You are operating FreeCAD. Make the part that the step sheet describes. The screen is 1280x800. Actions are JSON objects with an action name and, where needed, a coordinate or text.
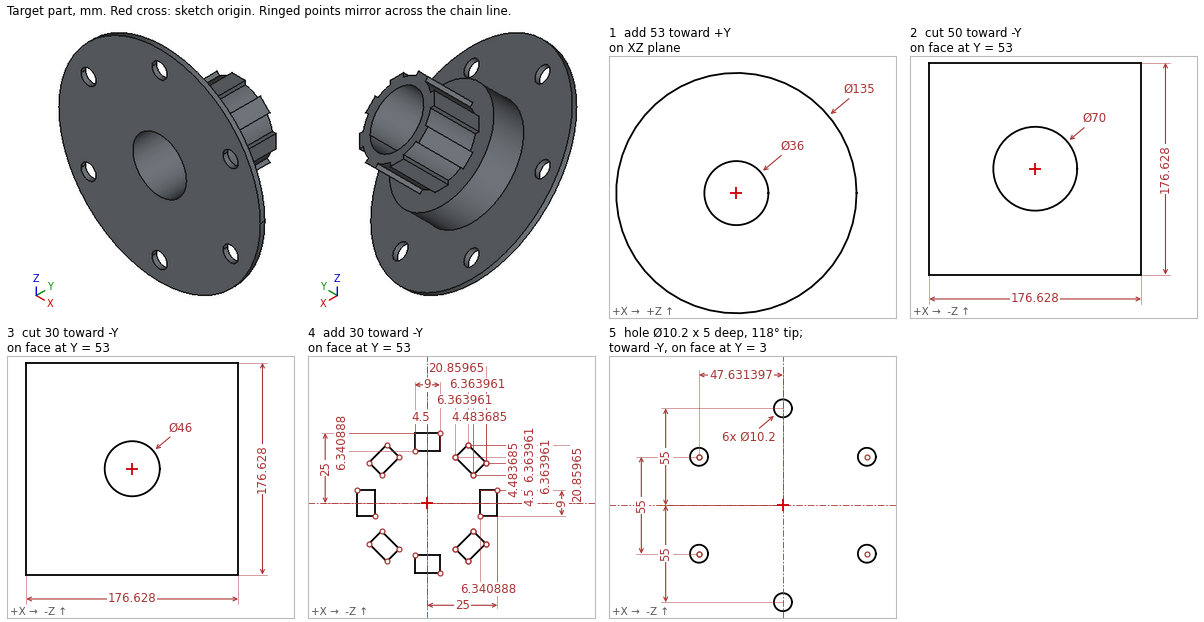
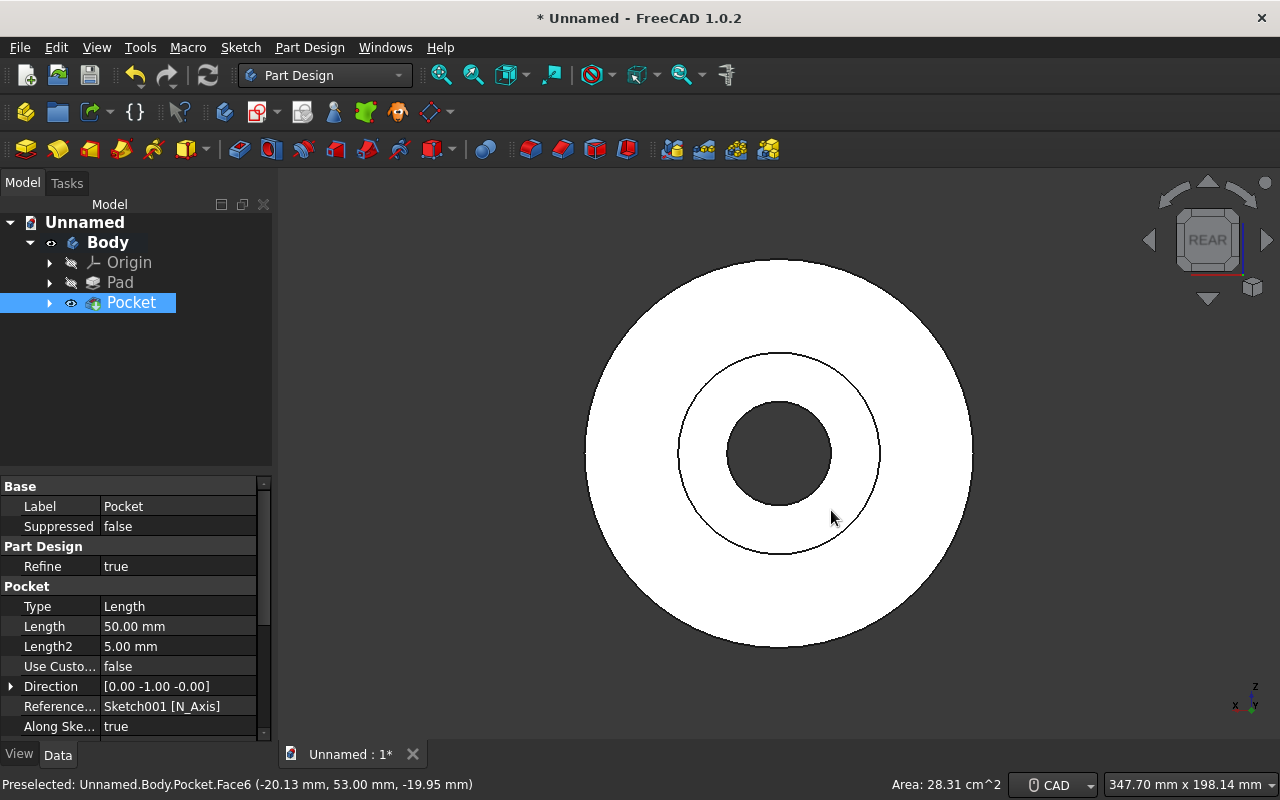
{"action": "left_click", "coordinate": [258, 112]}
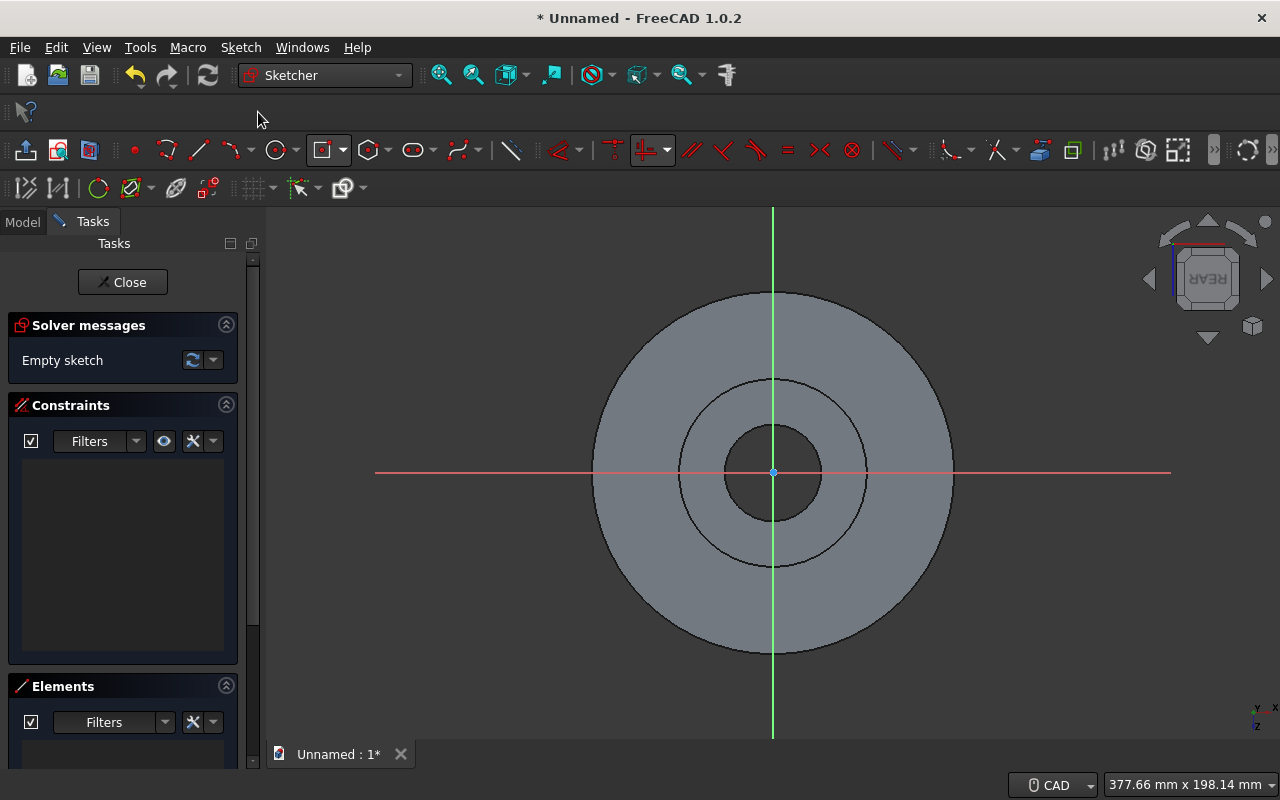
{"action": "scroll", "coordinate": [565, 473], "scroll_direction": "down", "scroll_amount": 2}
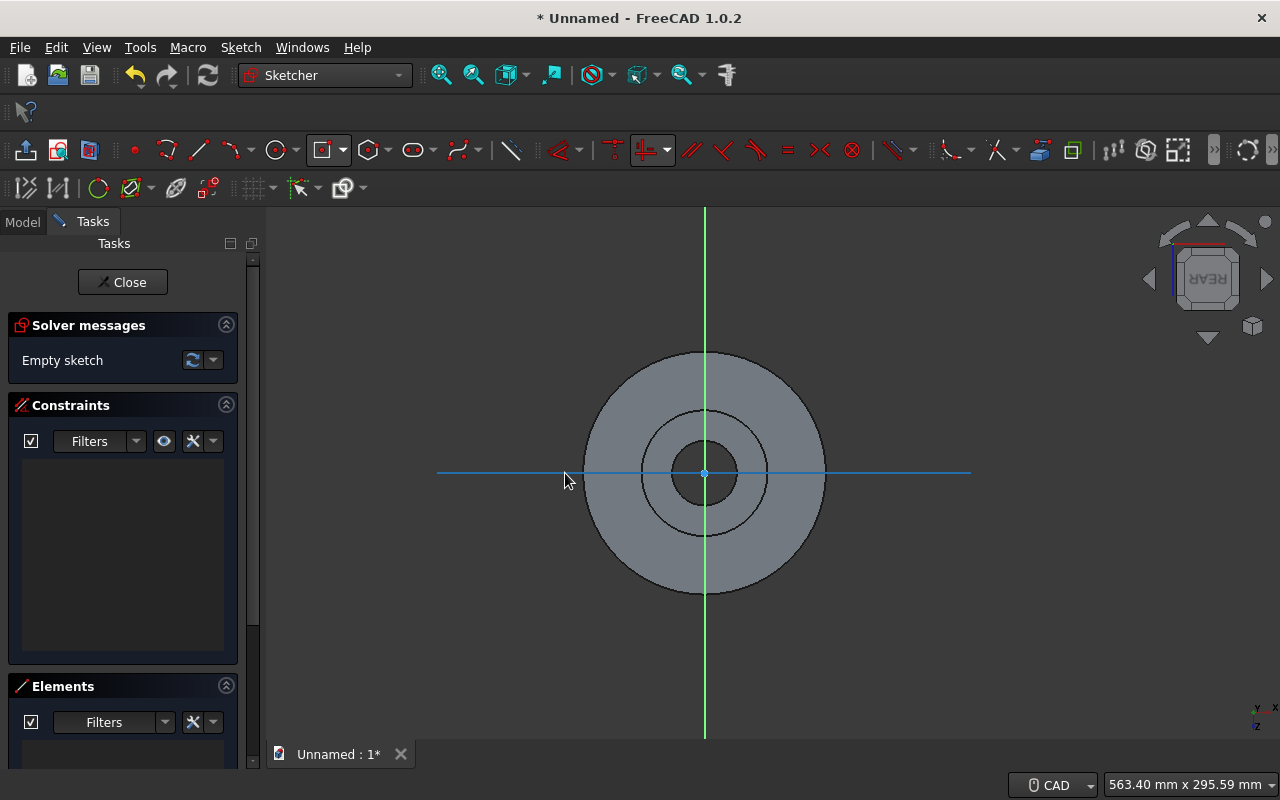
{"action": "left_click", "coordinate": [322, 150]}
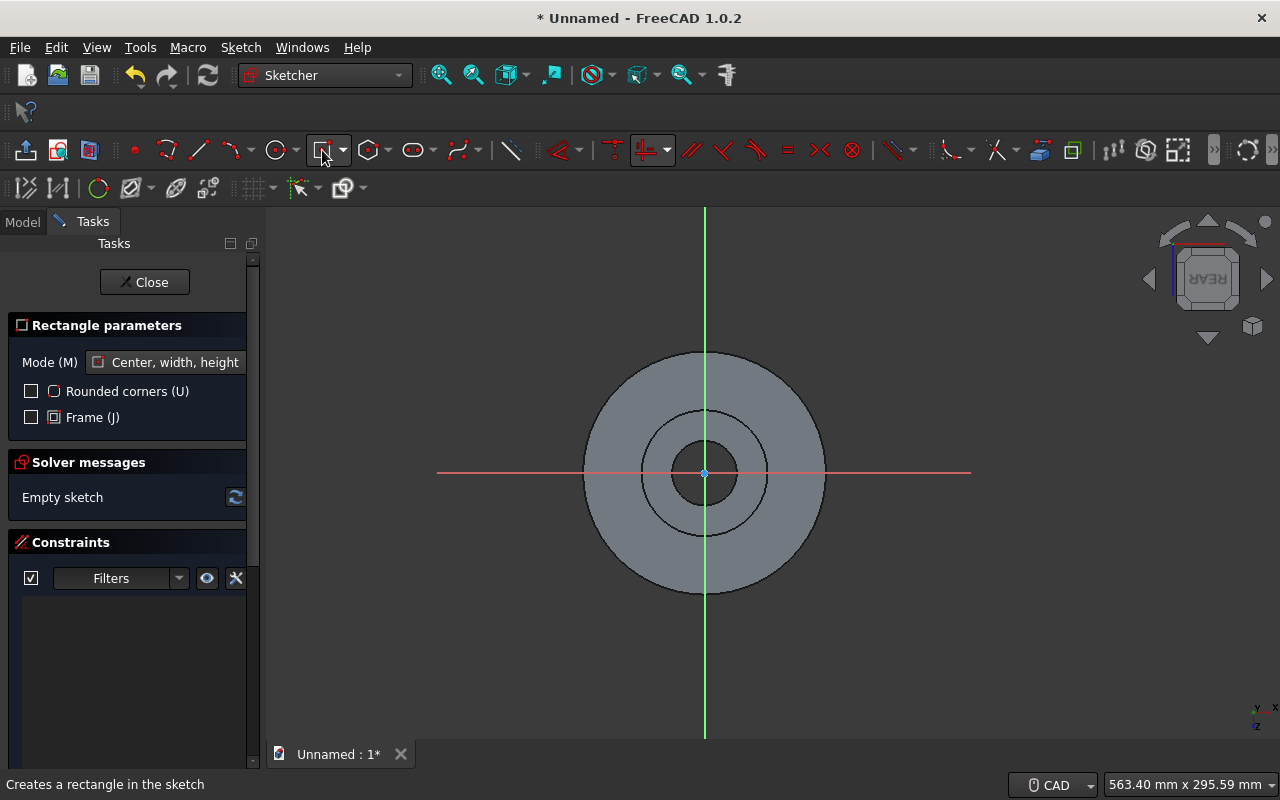
{"action": "left_click", "coordinate": [705, 473]}
{"action": "left_click", "coordinate": [863, 314]}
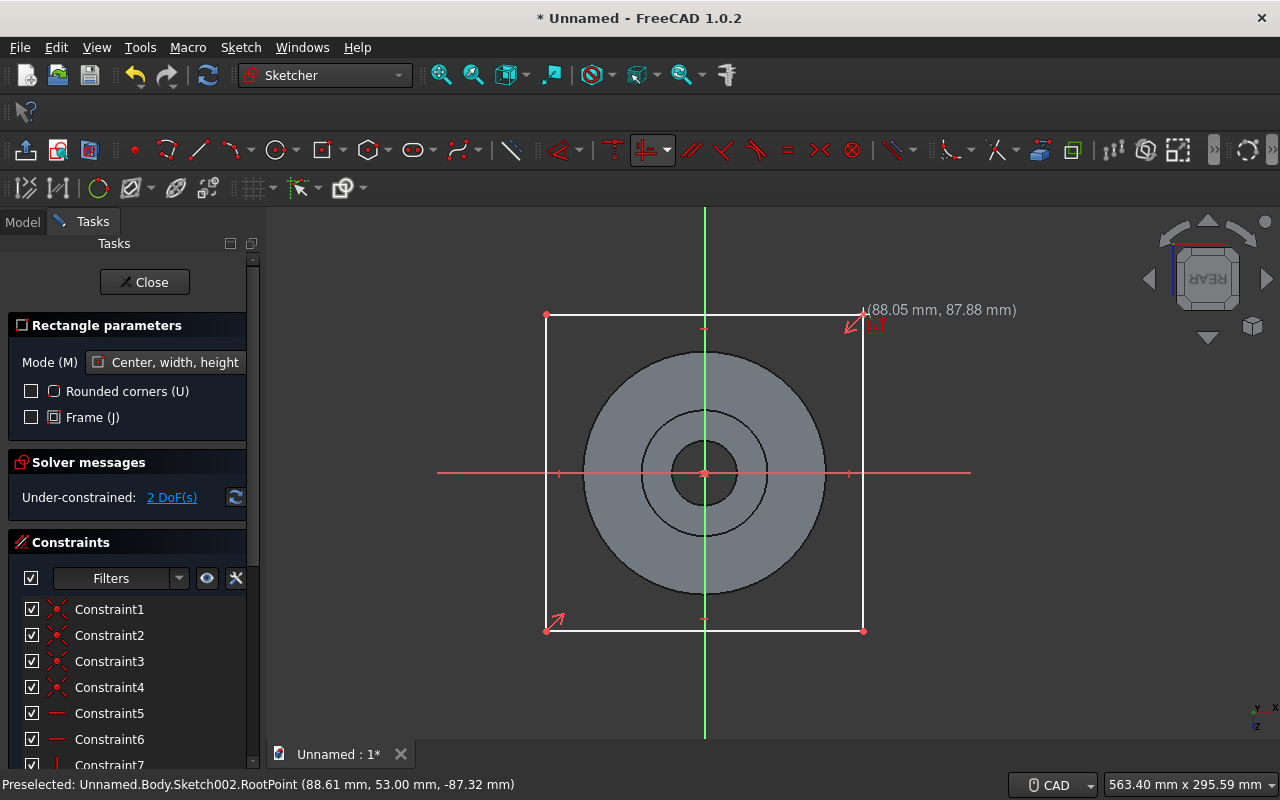
{"action": "left_click", "coordinate": [276, 150]}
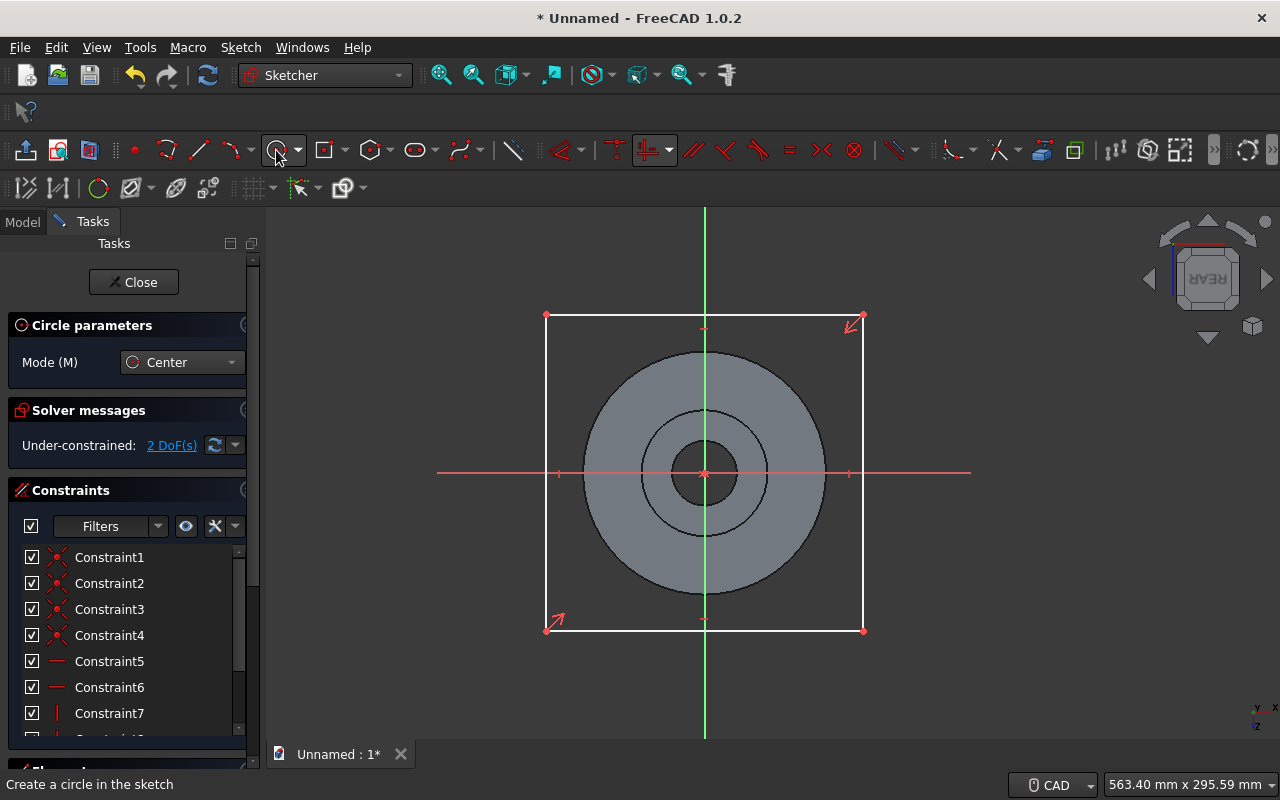
{"action": "left_click", "coordinate": [705, 473]}
{"action": "left_click", "coordinate": [734, 444]}
{"action": "key", "text": "Escape"}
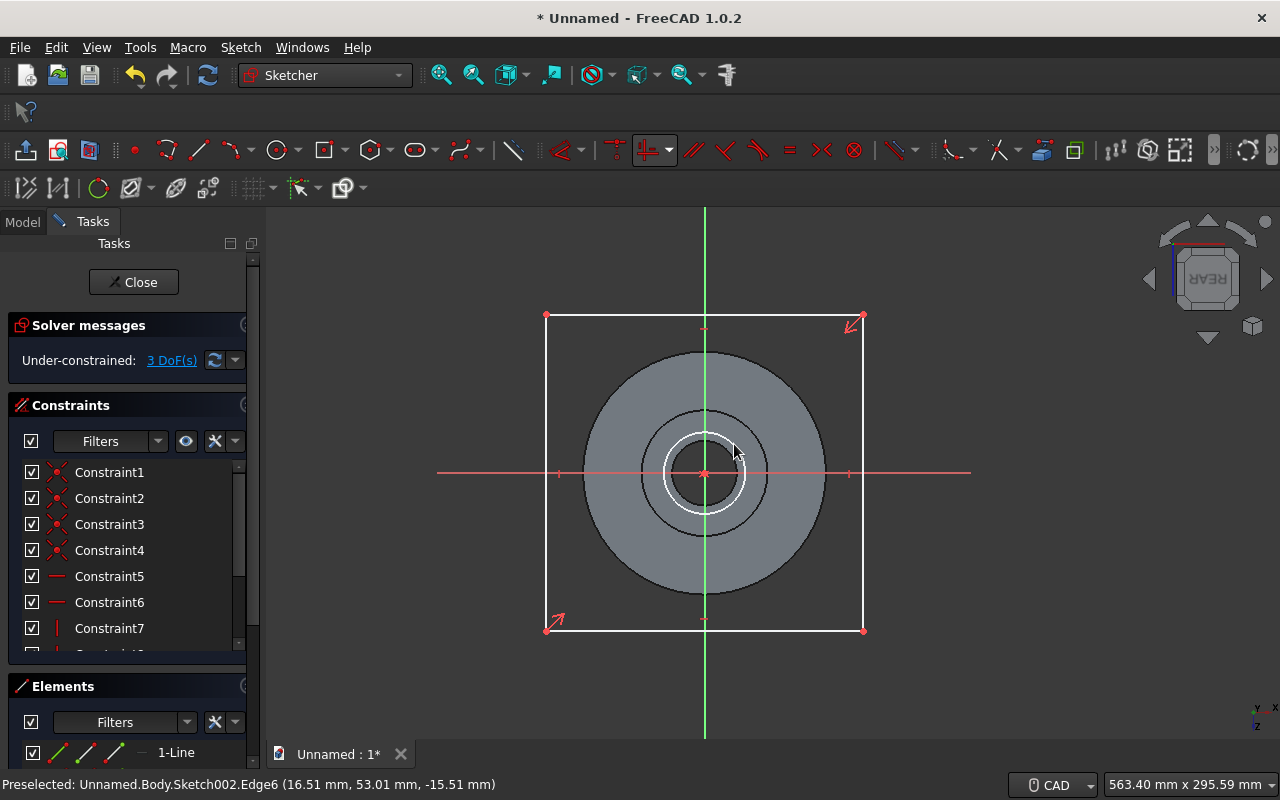
{"action": "left_click", "coordinate": [560, 150]}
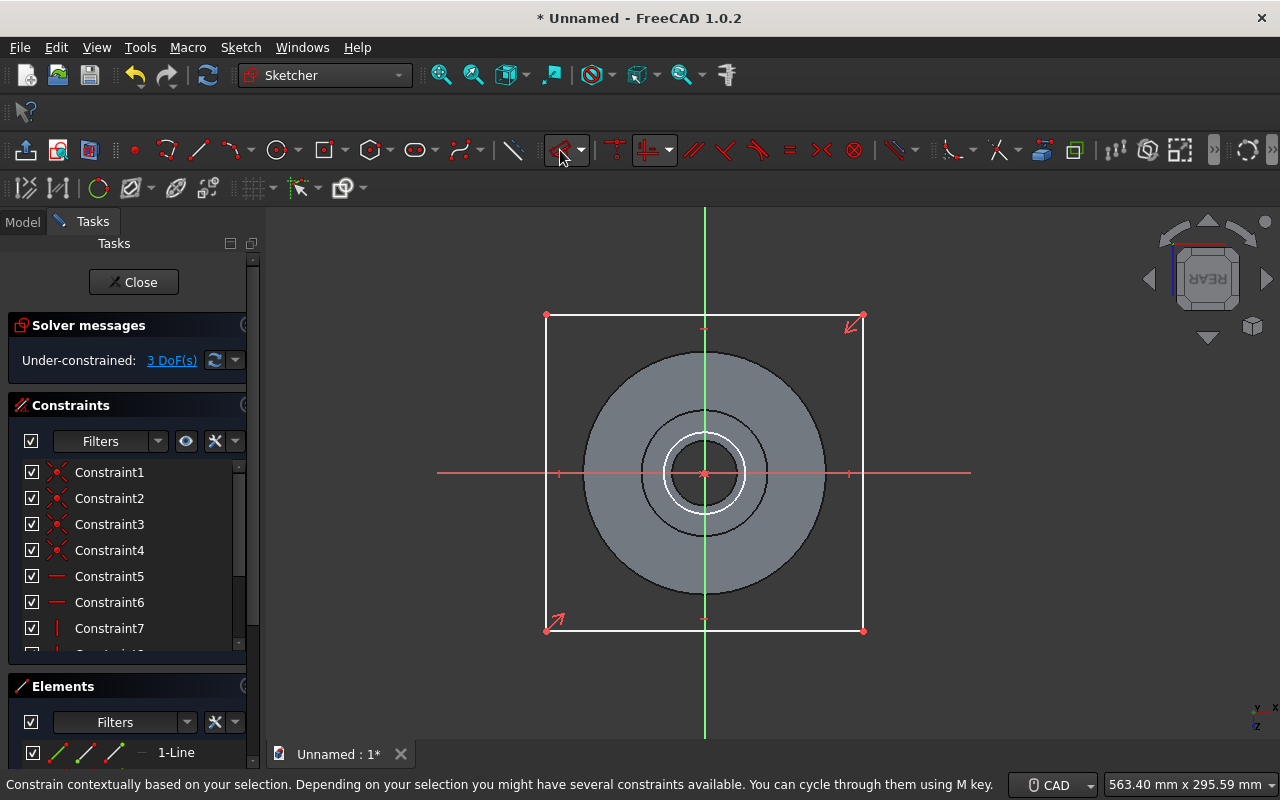
{"action": "left_click", "coordinate": [733, 444]}
{"action": "left_click", "coordinate": [755, 421]}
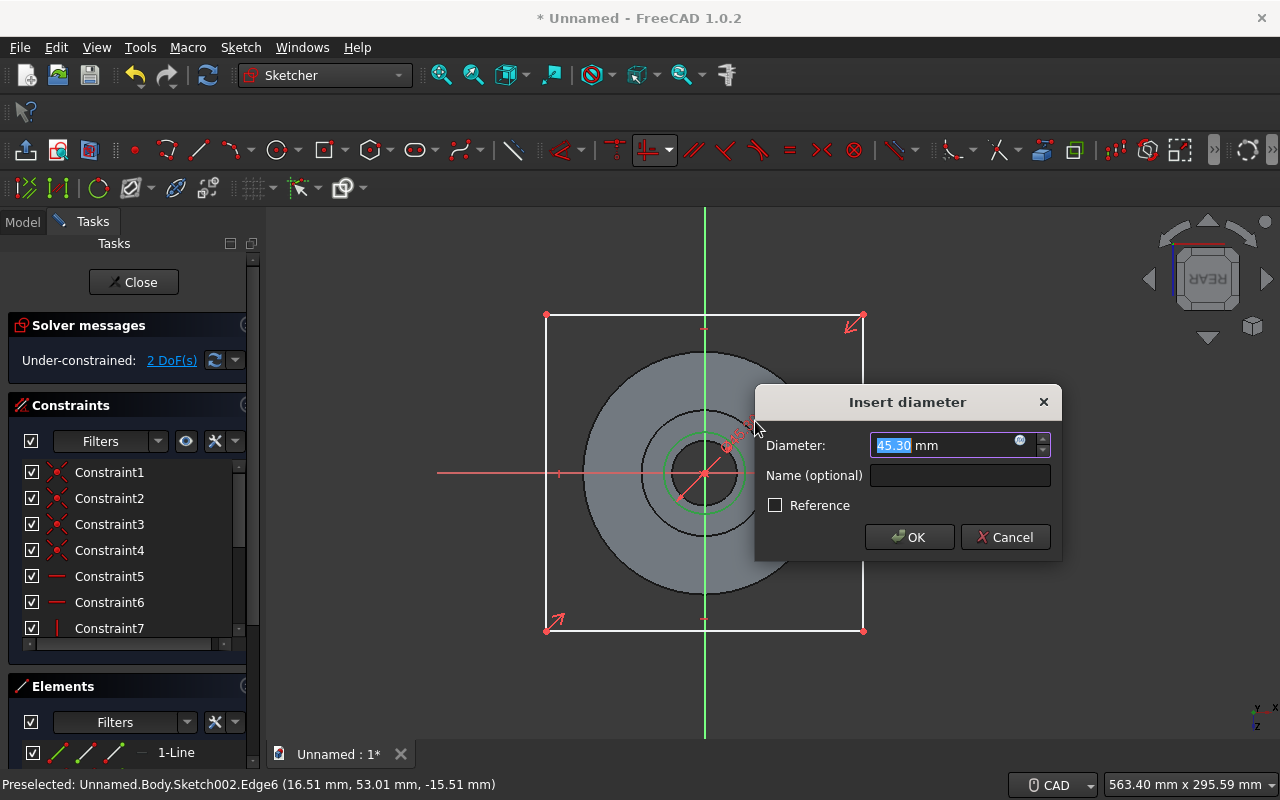
{"action": "type", "text": "46"}
{"action": "key", "text": "Return"}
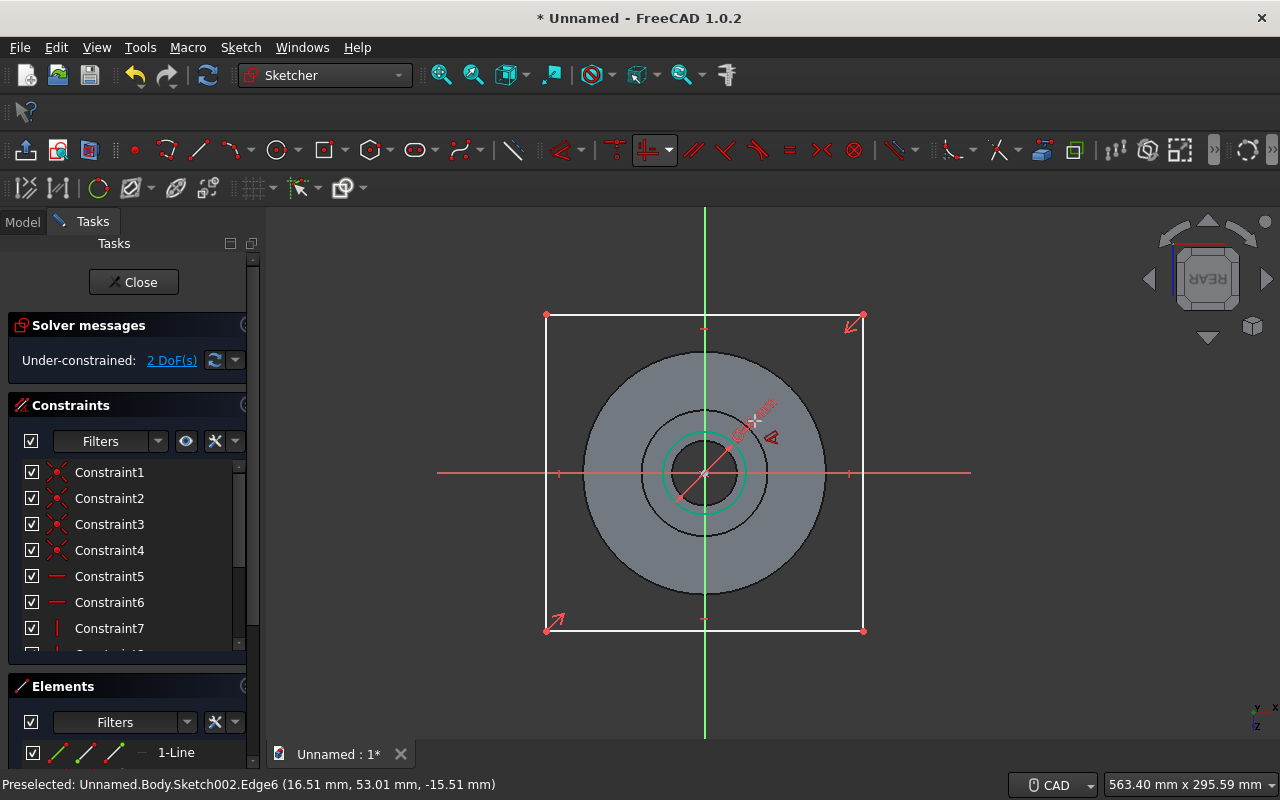
{"action": "left_click", "coordinate": [641, 631]}
{"action": "left_click", "coordinate": [632, 665]}